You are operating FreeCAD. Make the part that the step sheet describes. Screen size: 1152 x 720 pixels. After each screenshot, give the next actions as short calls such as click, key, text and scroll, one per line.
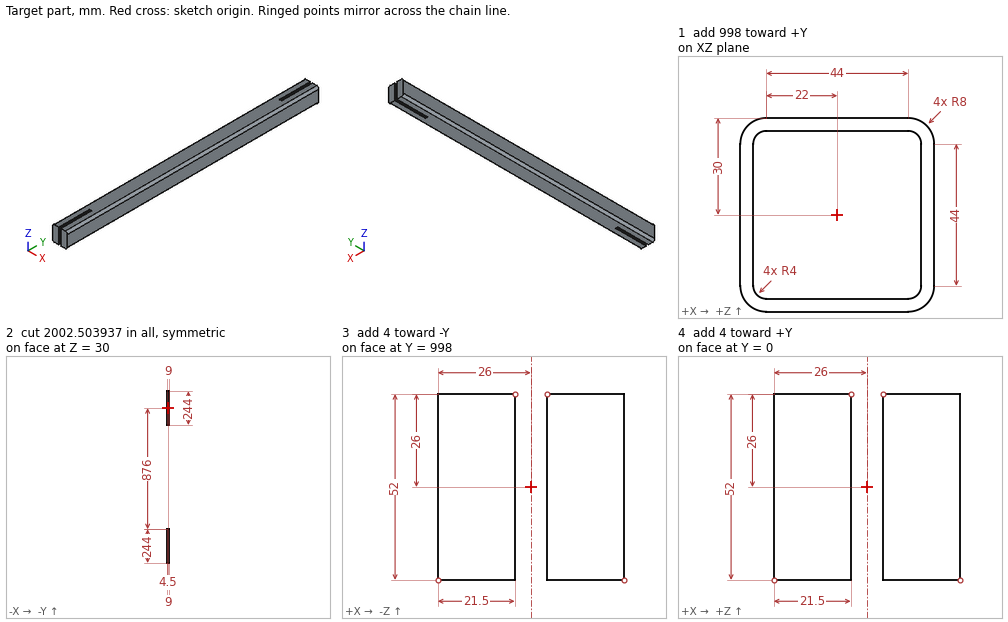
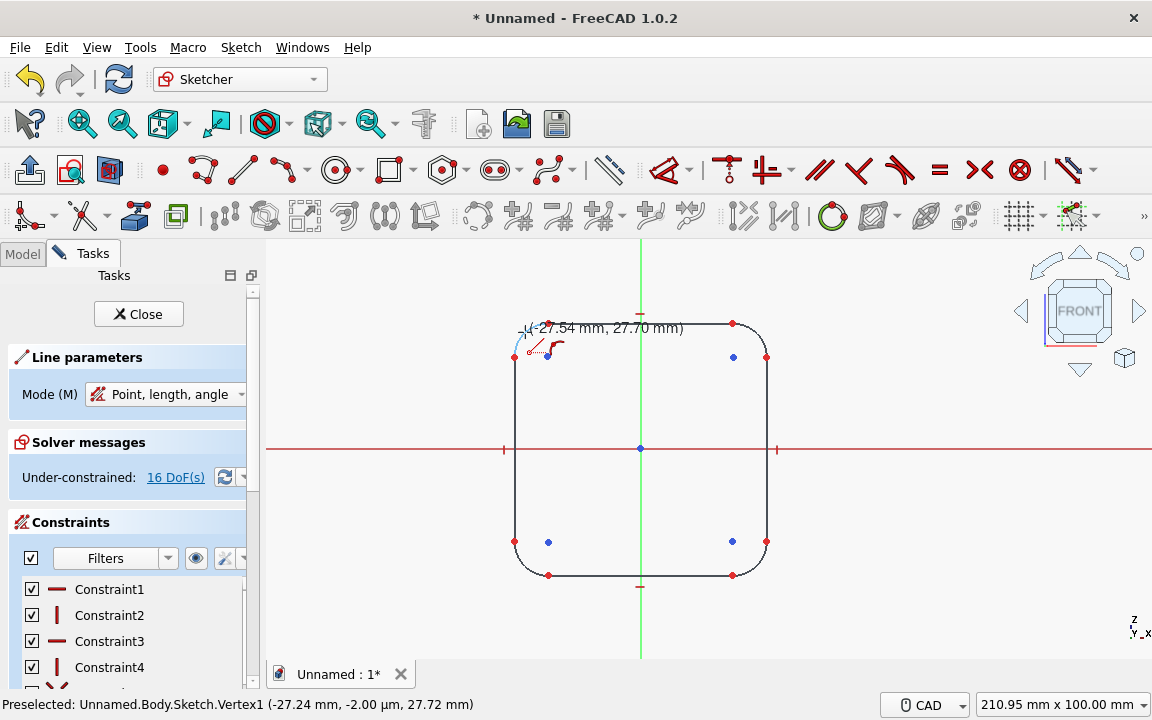
click(548, 558)
click(733, 558)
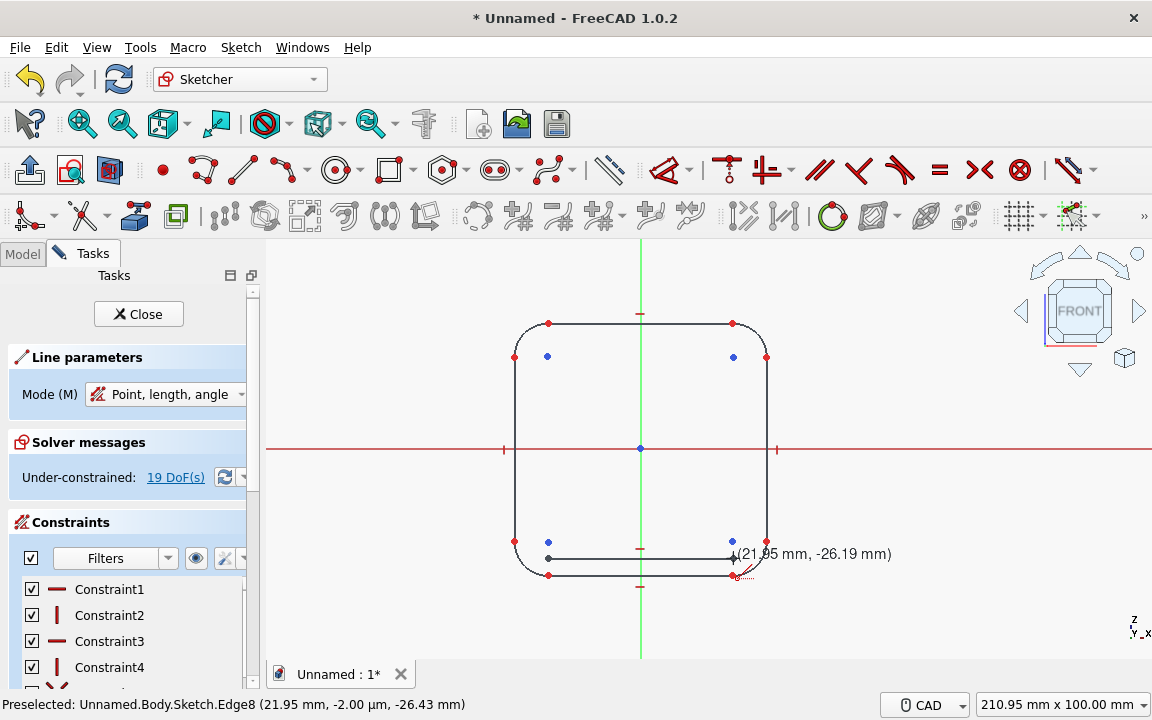
click(750, 541)
click(750, 357)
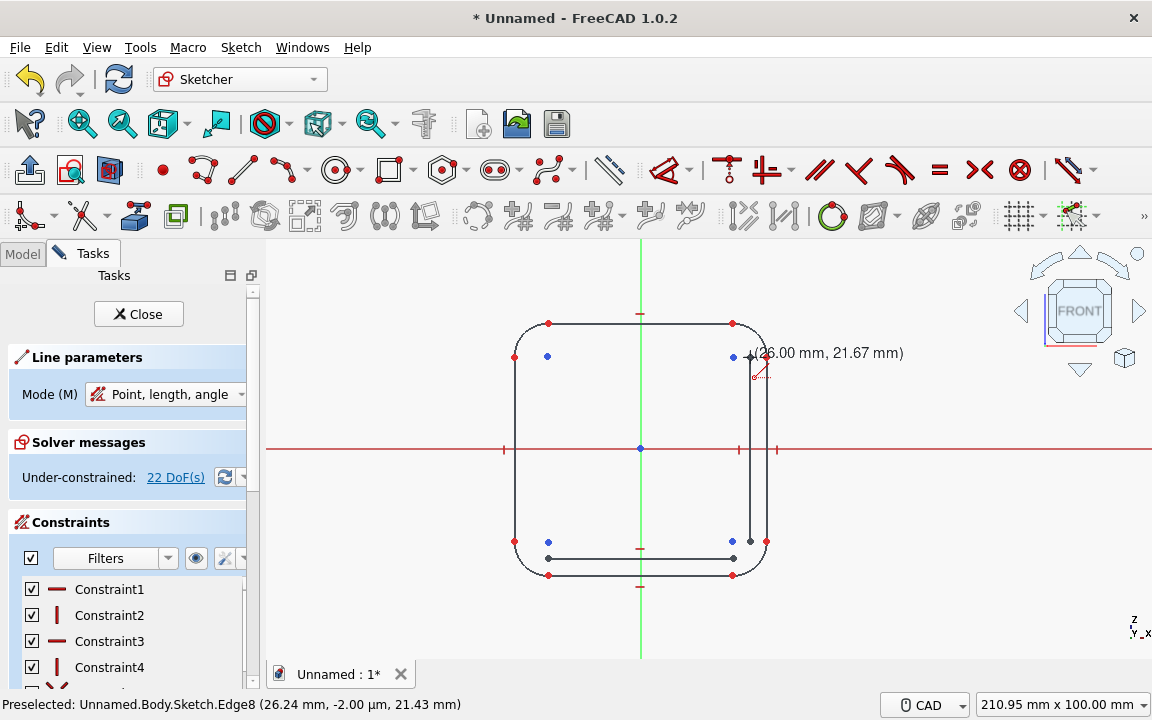
click(733, 340)
click(548, 340)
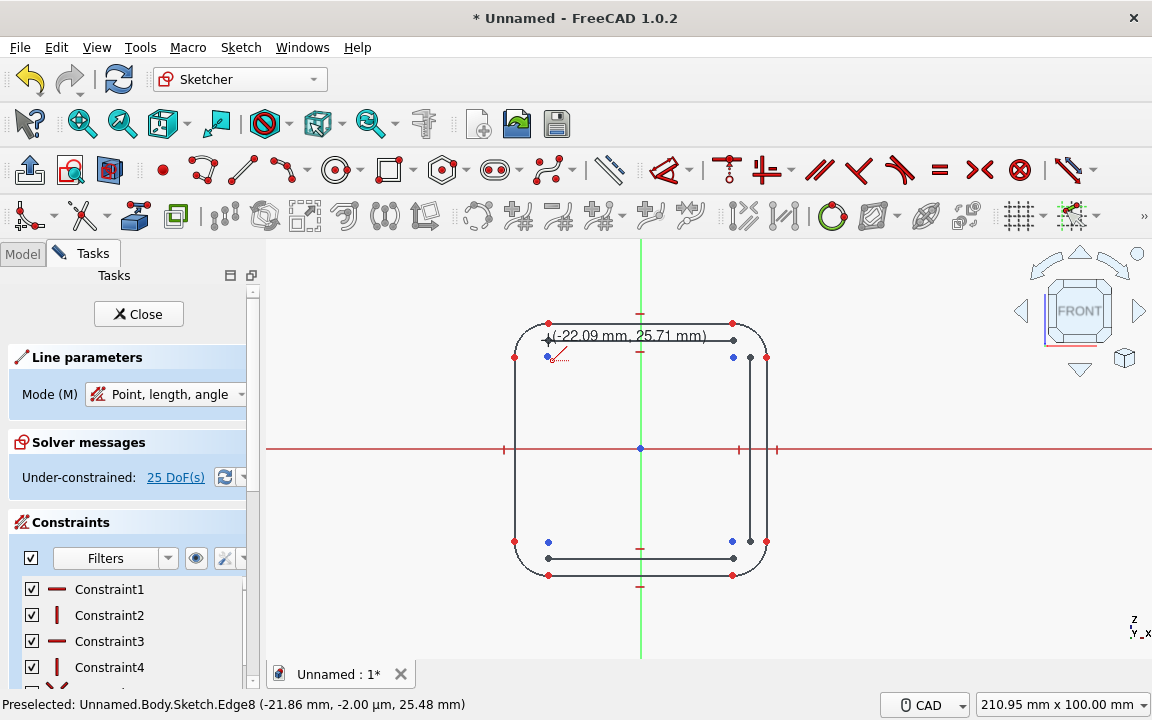
click(532, 357)
click(532, 541)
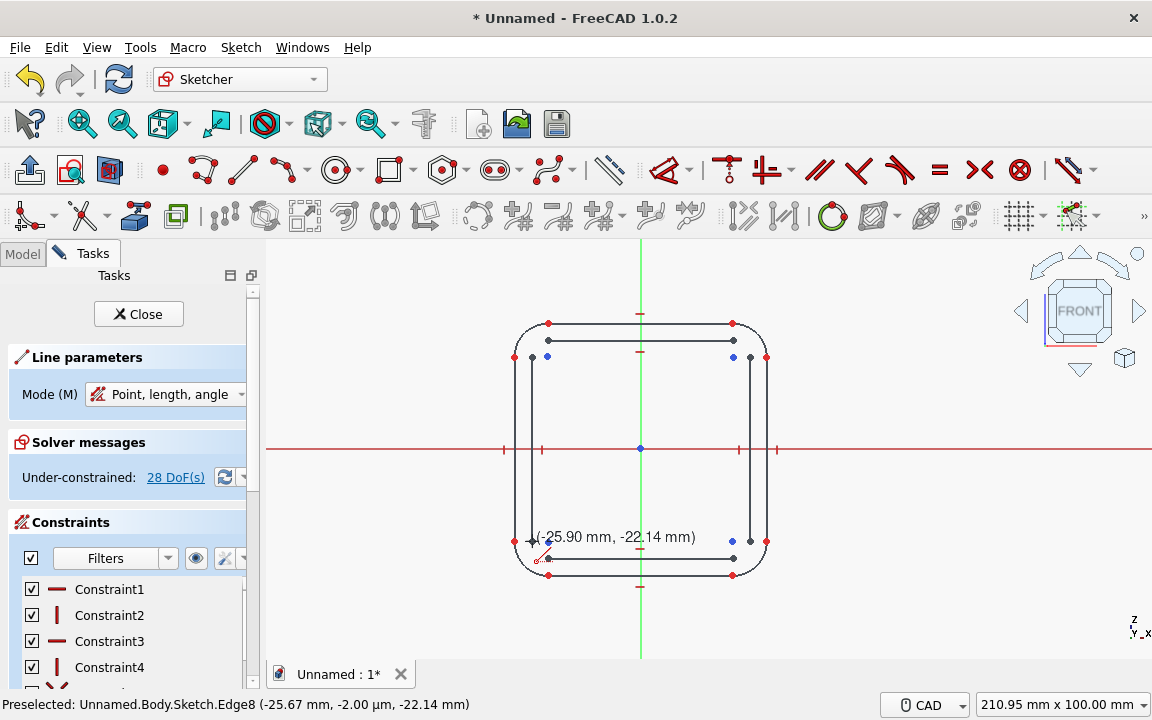
click(284, 170)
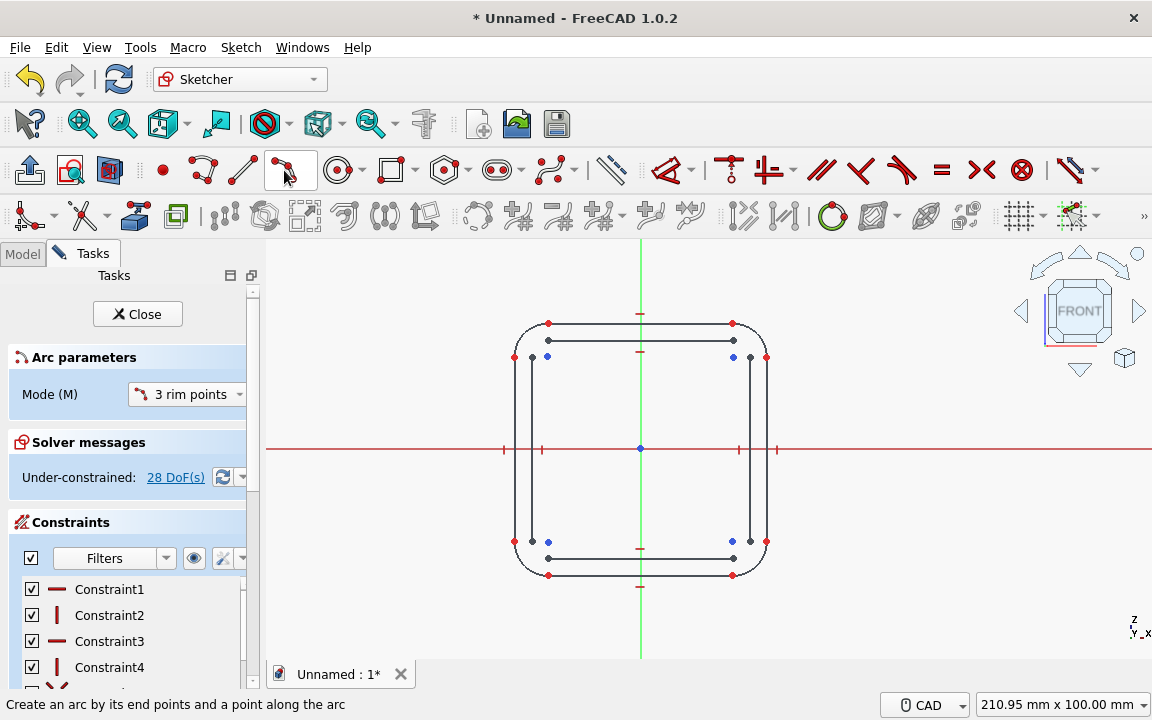
click(733, 559)
click(750, 542)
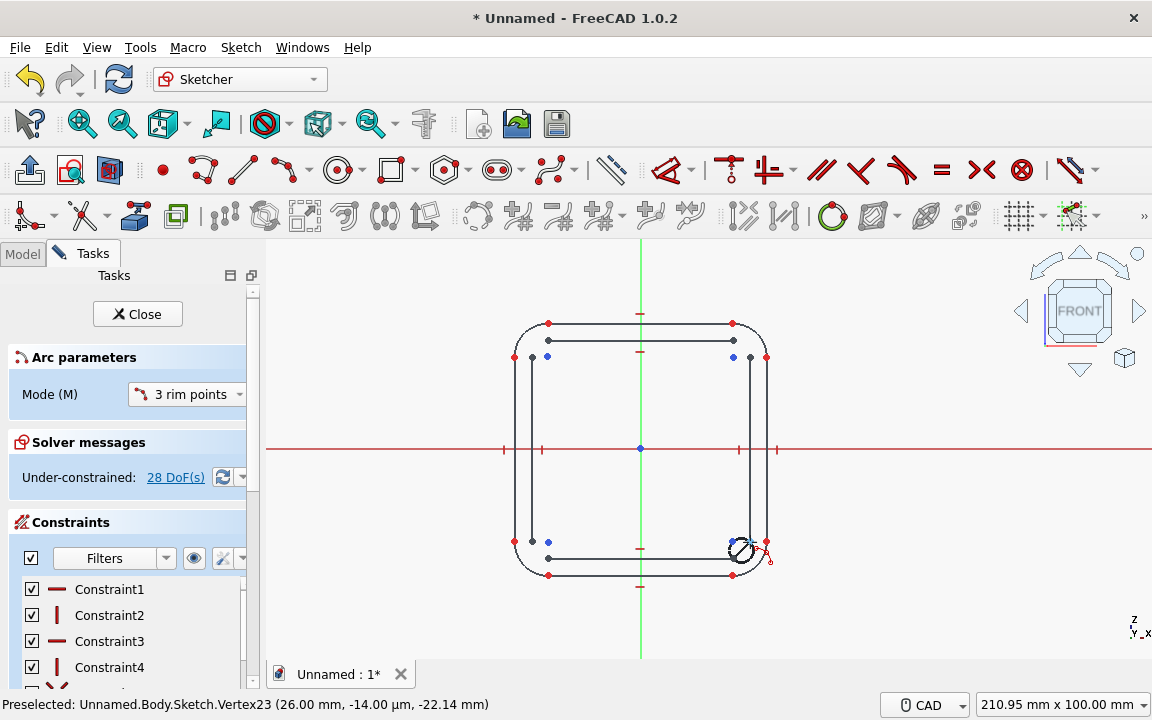
scroll(745, 553, up, 6)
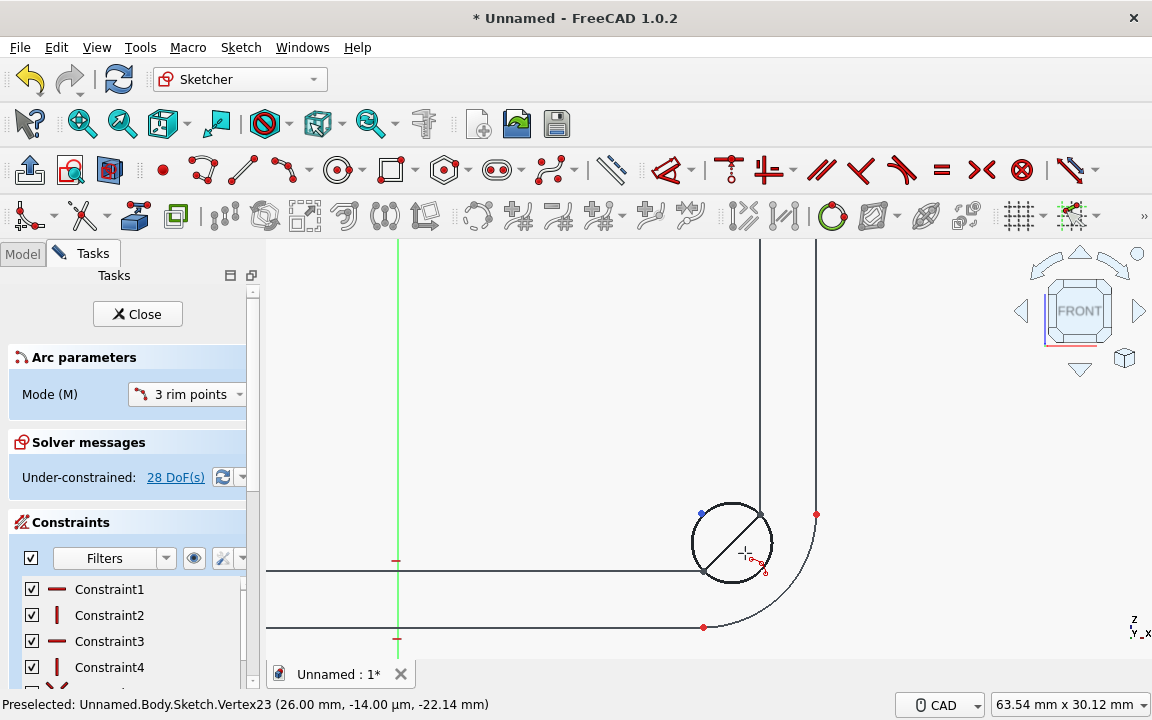
click(744, 552)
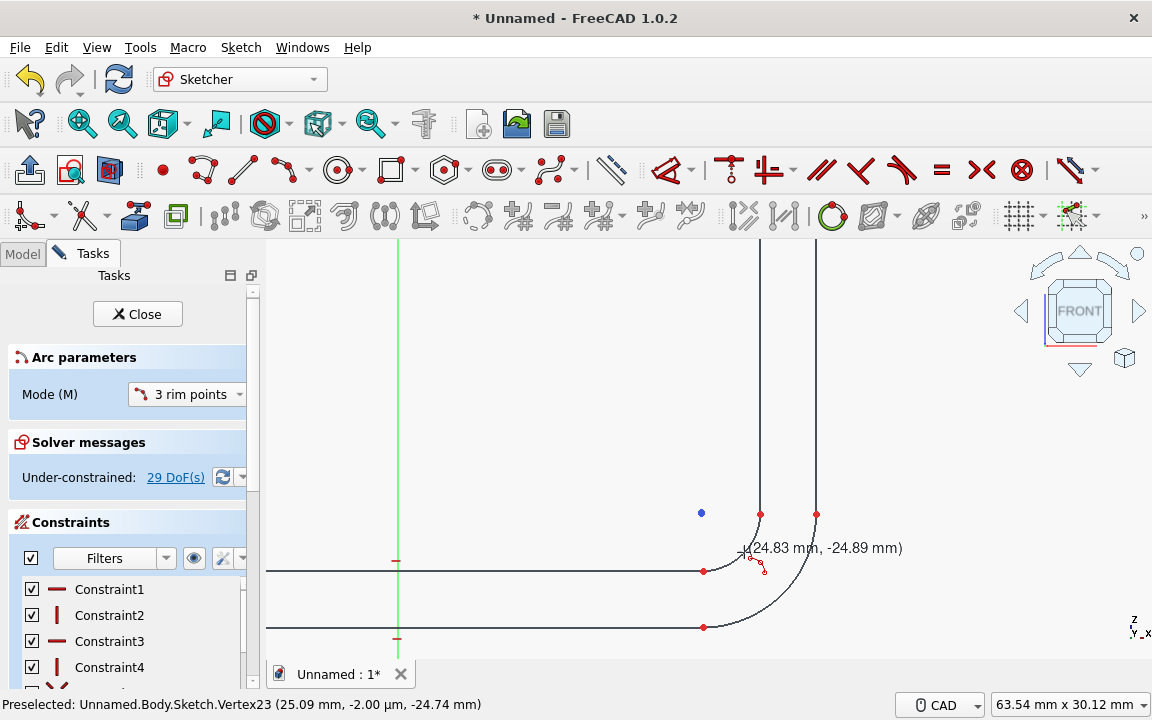
scroll(745, 554, down, 6)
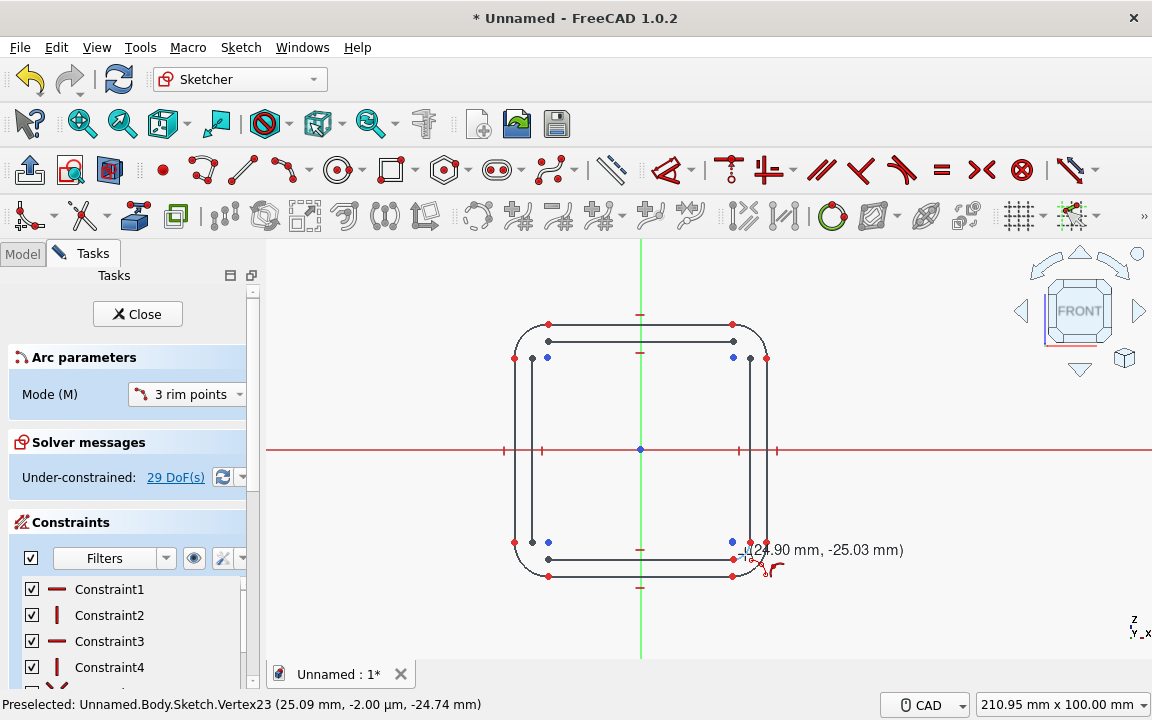
click(750, 359)
click(733, 342)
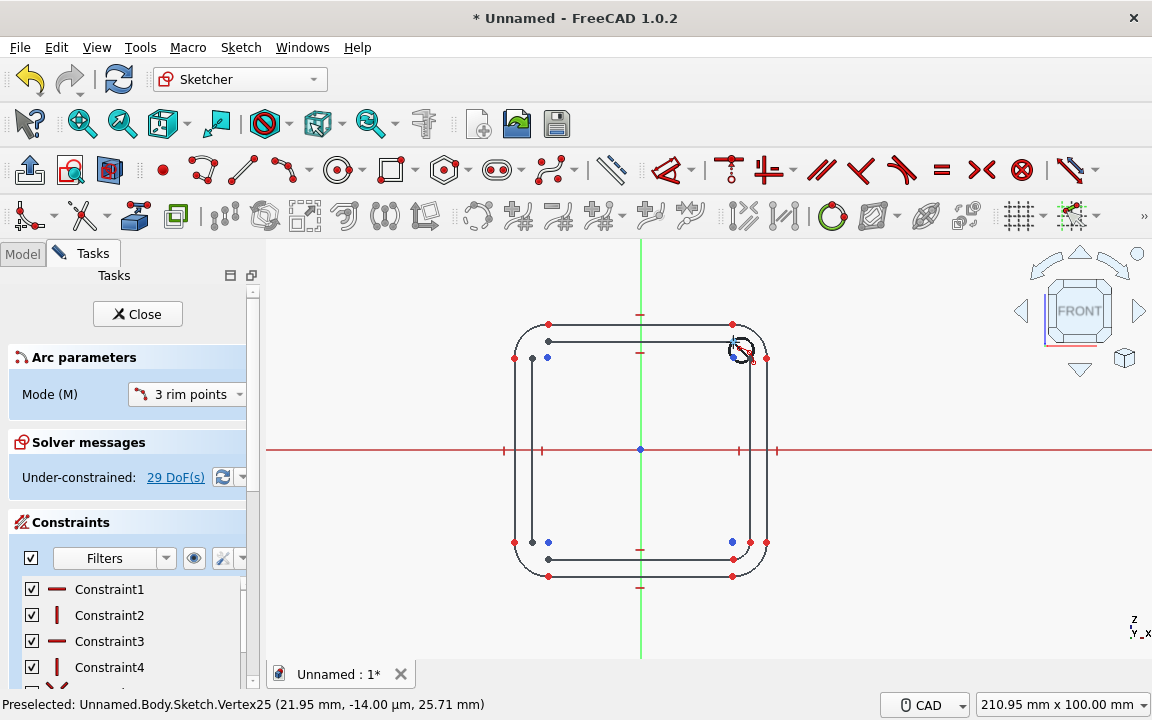
scroll(745, 345, up, 6)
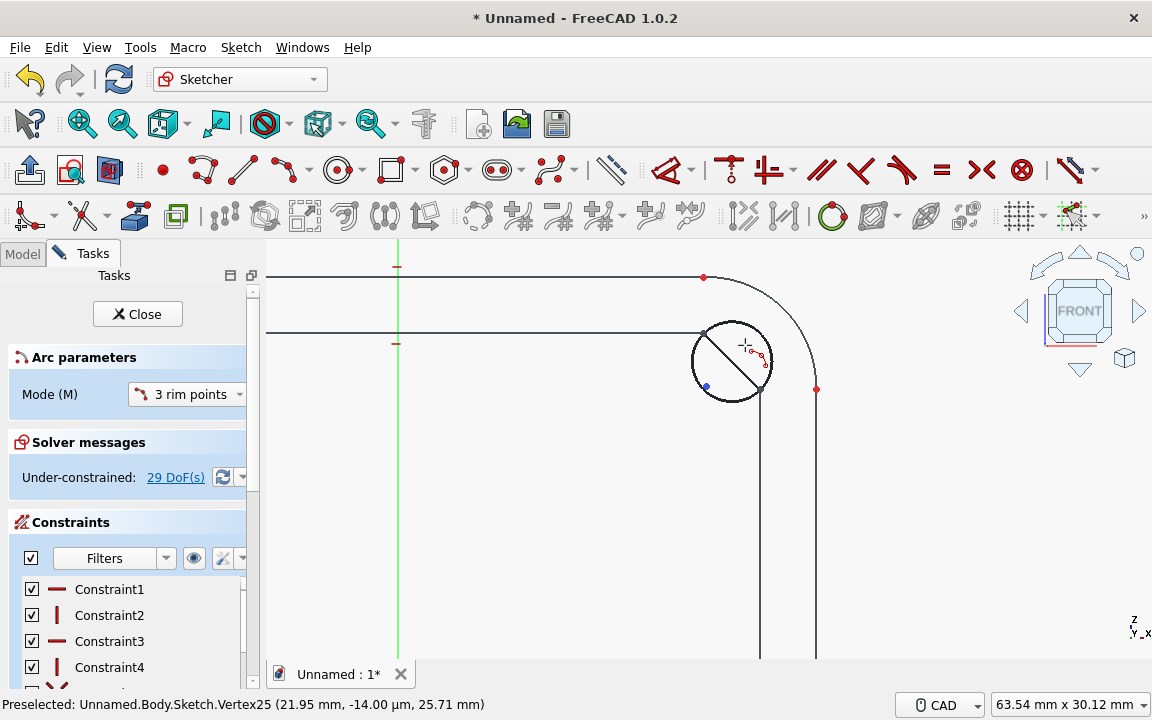
click(744, 346)